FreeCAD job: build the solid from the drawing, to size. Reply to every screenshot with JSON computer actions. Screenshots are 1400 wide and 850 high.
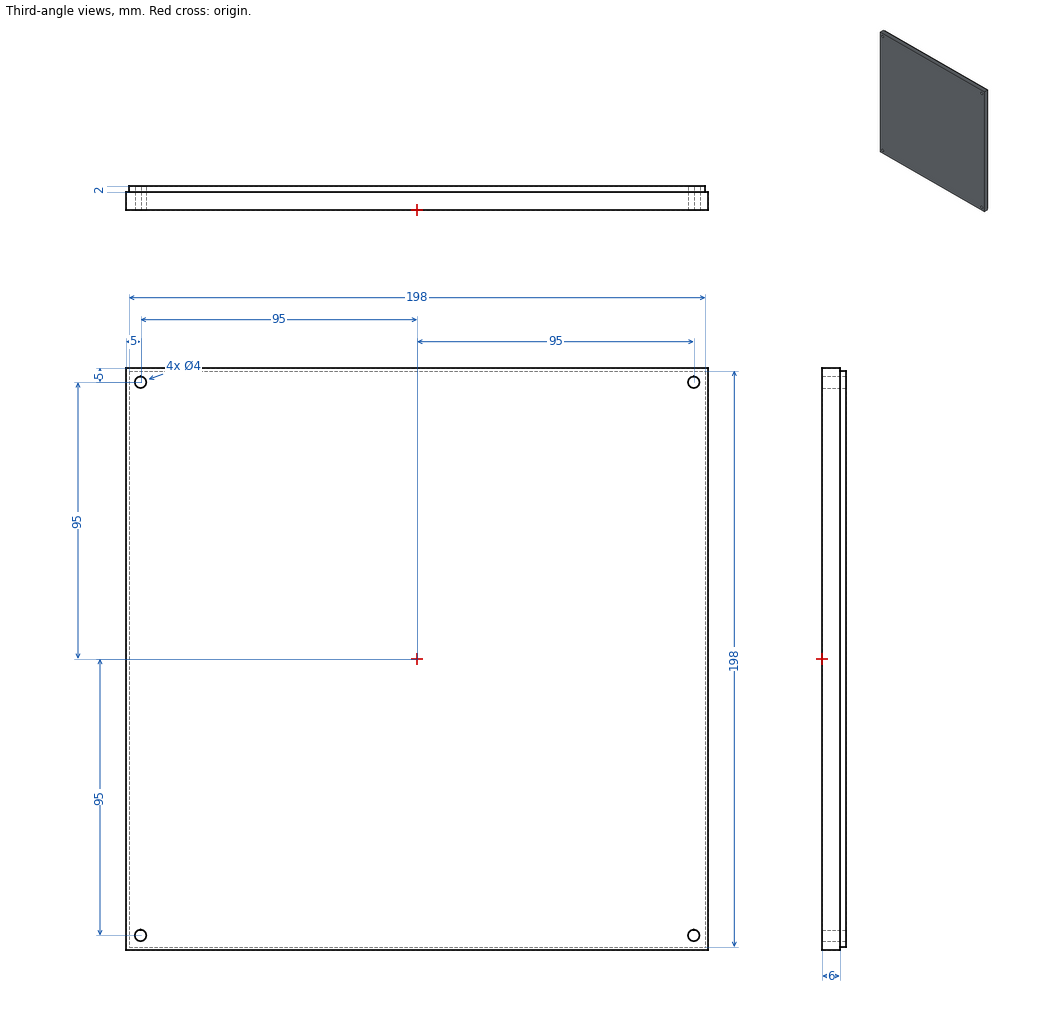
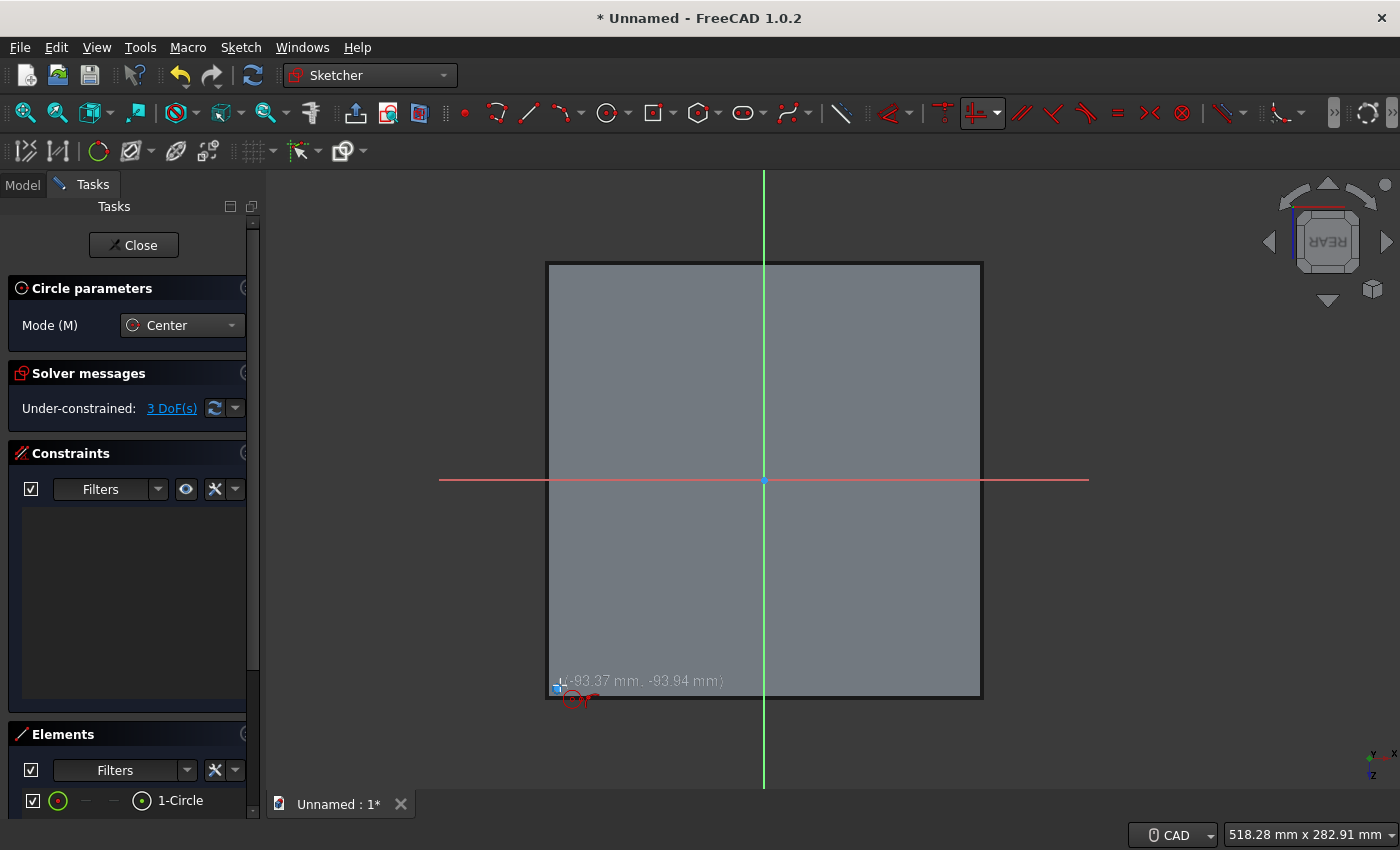
{"action": "scroll", "coordinate": [972, 688], "scroll_direction": "up", "scroll_amount": 9}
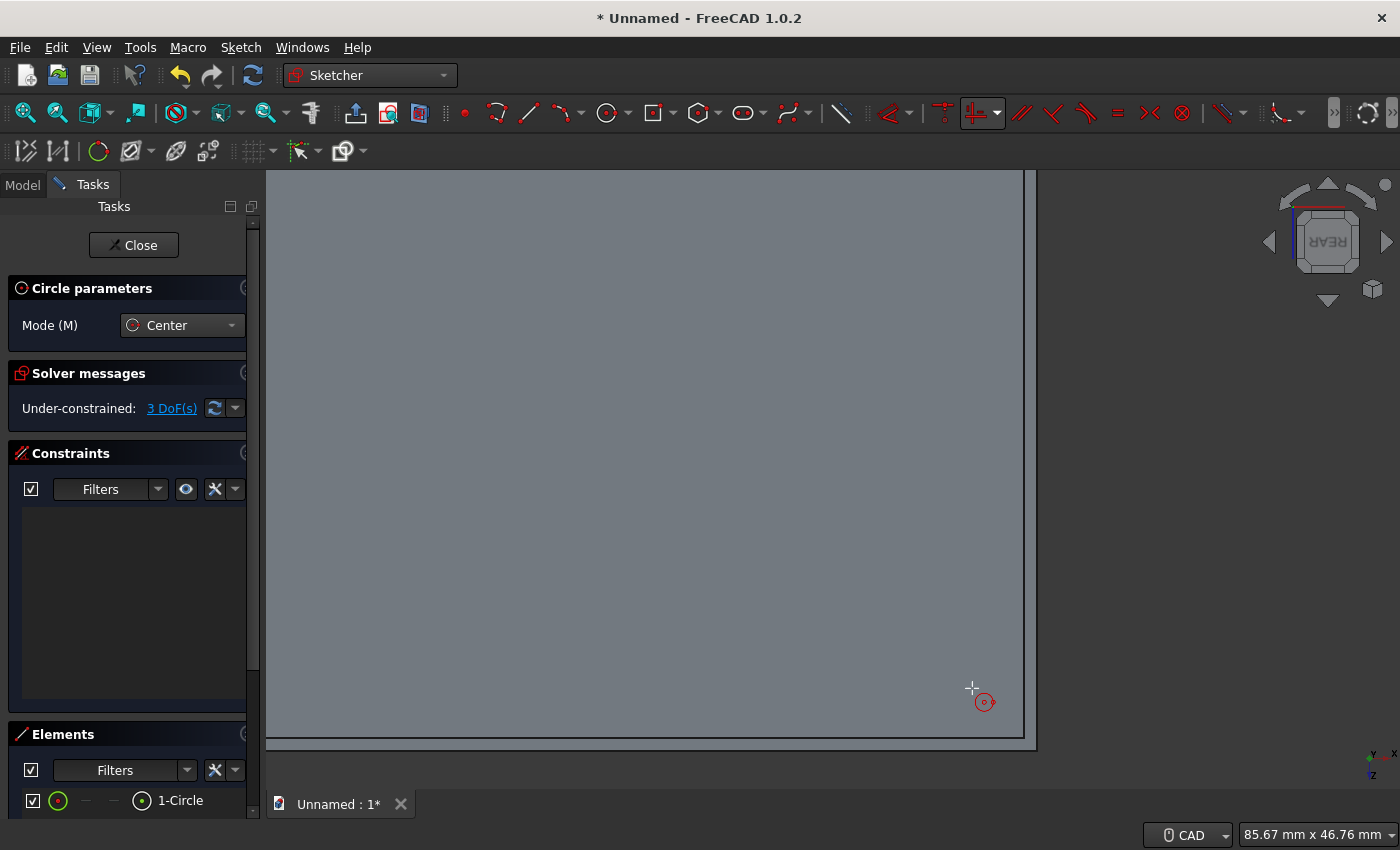
{"action": "scroll", "coordinate": [973, 688], "scroll_direction": "down", "scroll_amount": 9}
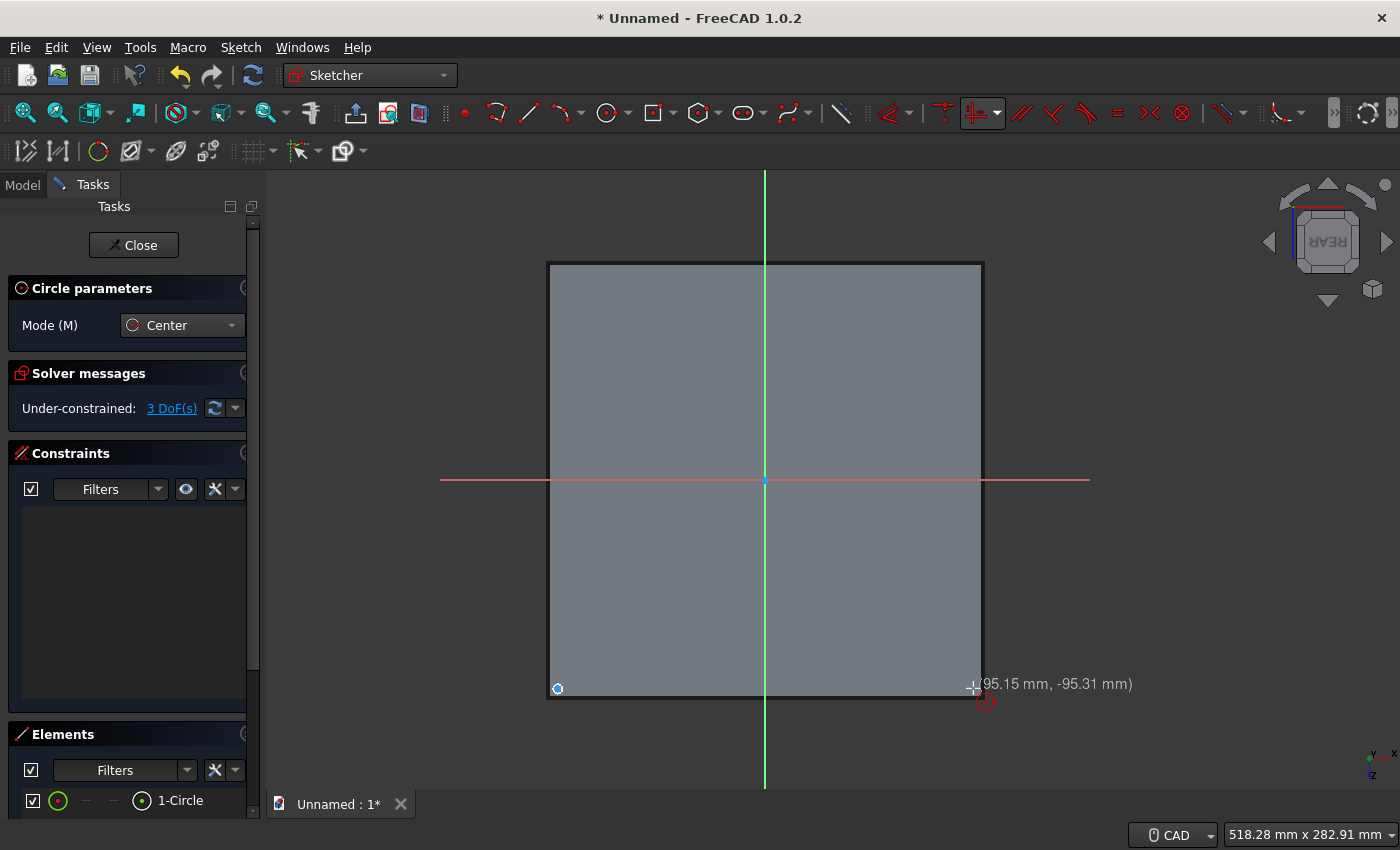
{"action": "left_click", "coordinate": [973, 688]}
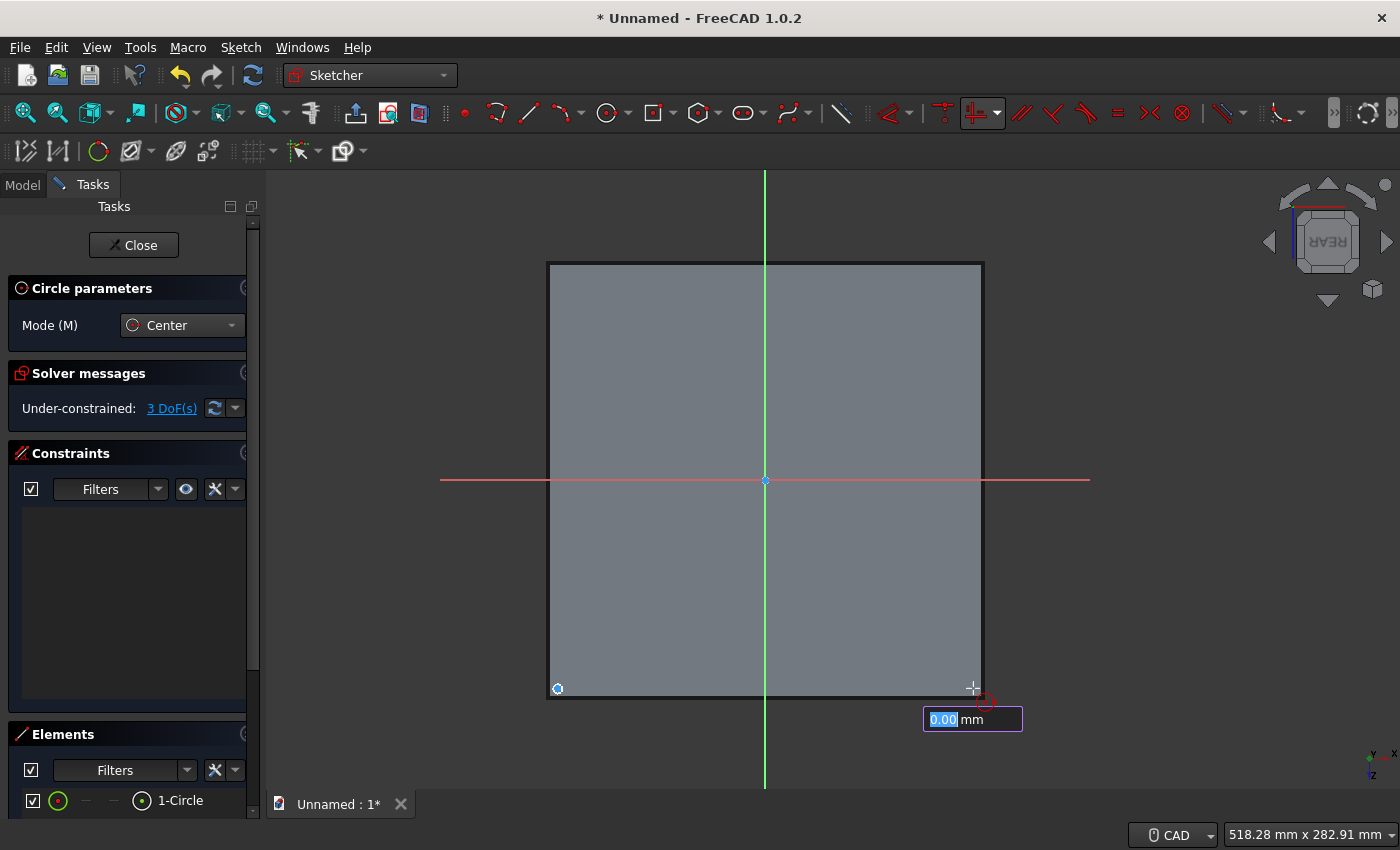
{"action": "scroll", "coordinate": [976, 685], "scroll_direction": "up", "scroll_amount": 7}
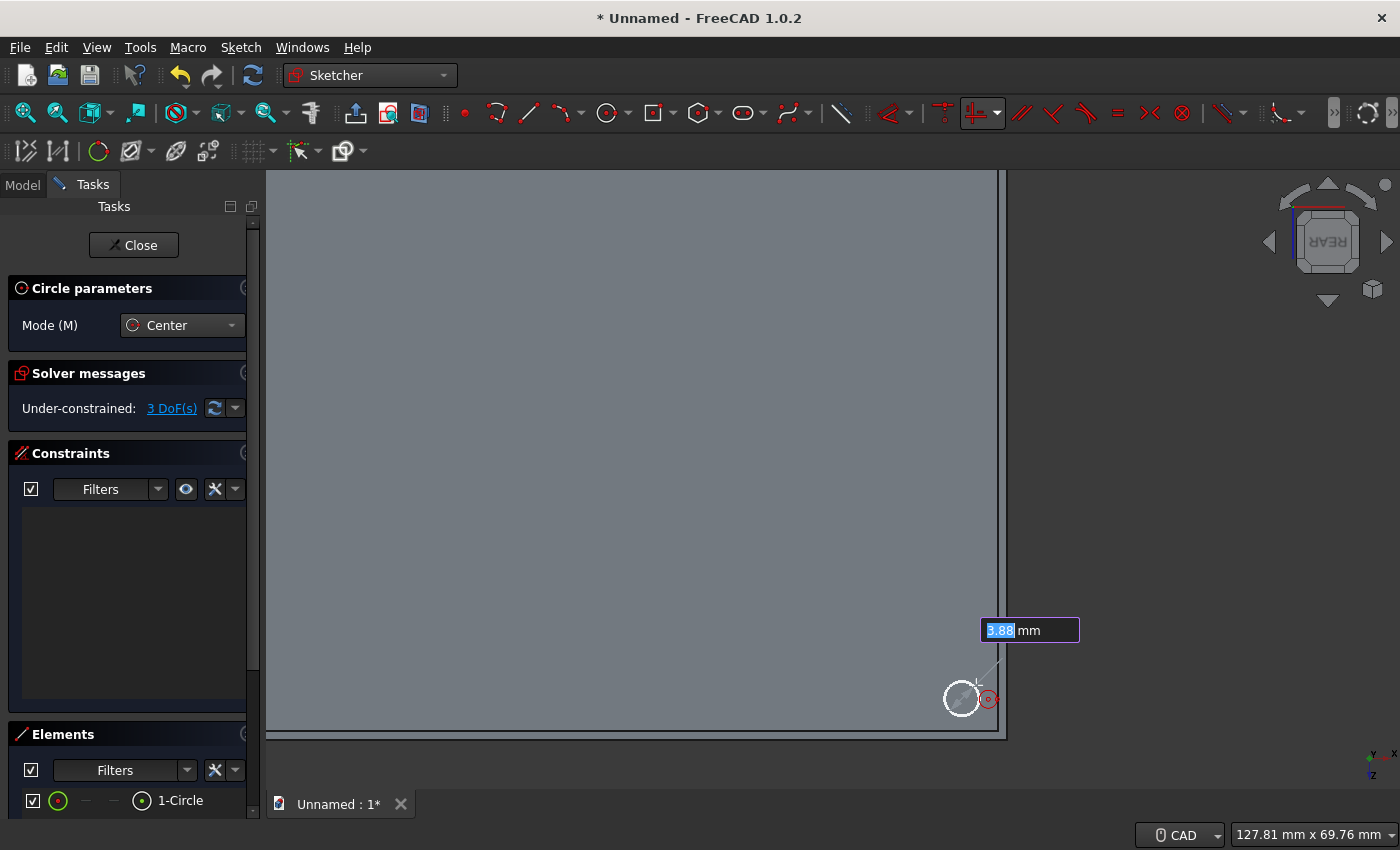
{"action": "left_click", "coordinate": [975, 683]}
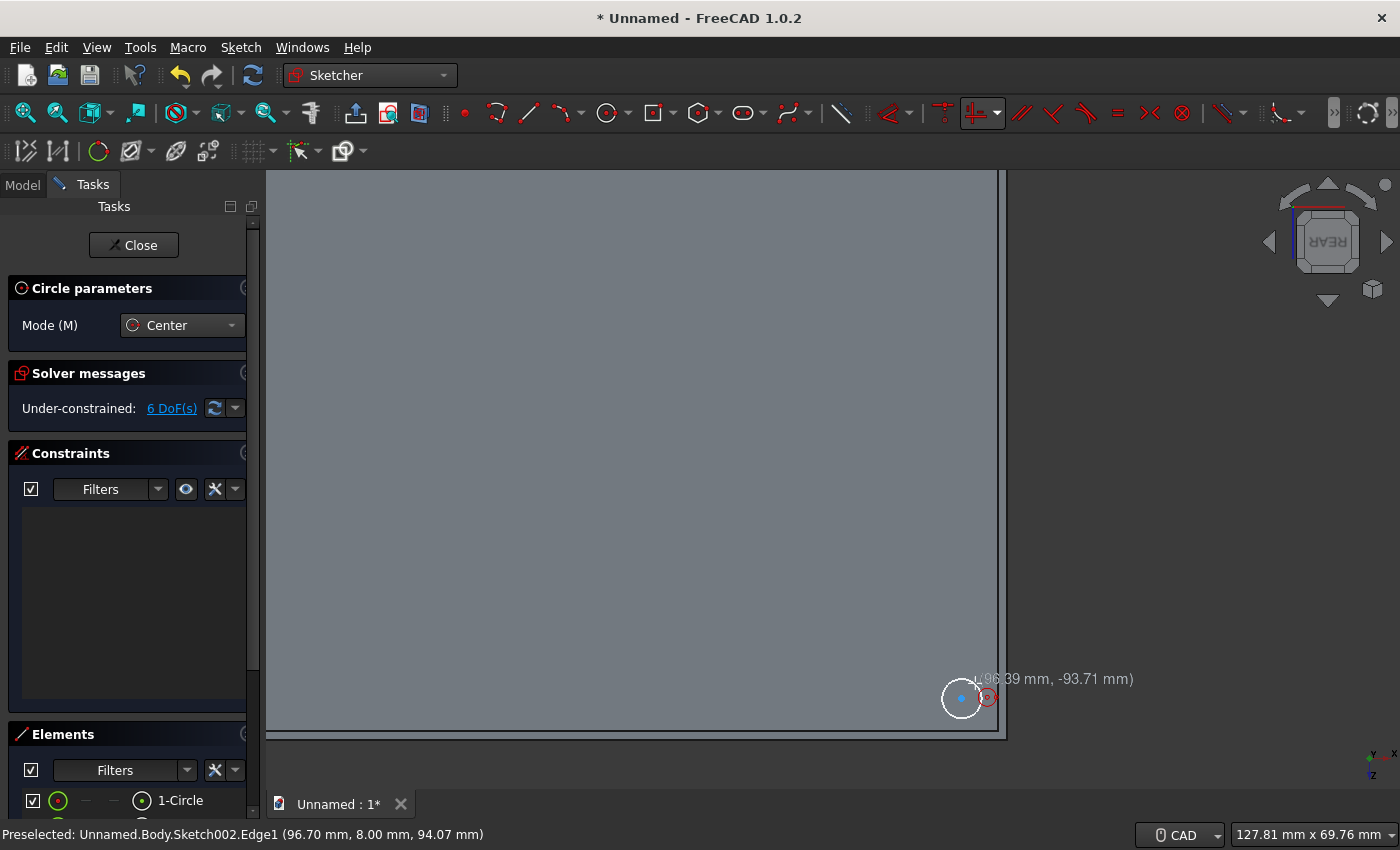
{"action": "scroll", "coordinate": [976, 685], "scroll_direction": "down", "scroll_amount": 7}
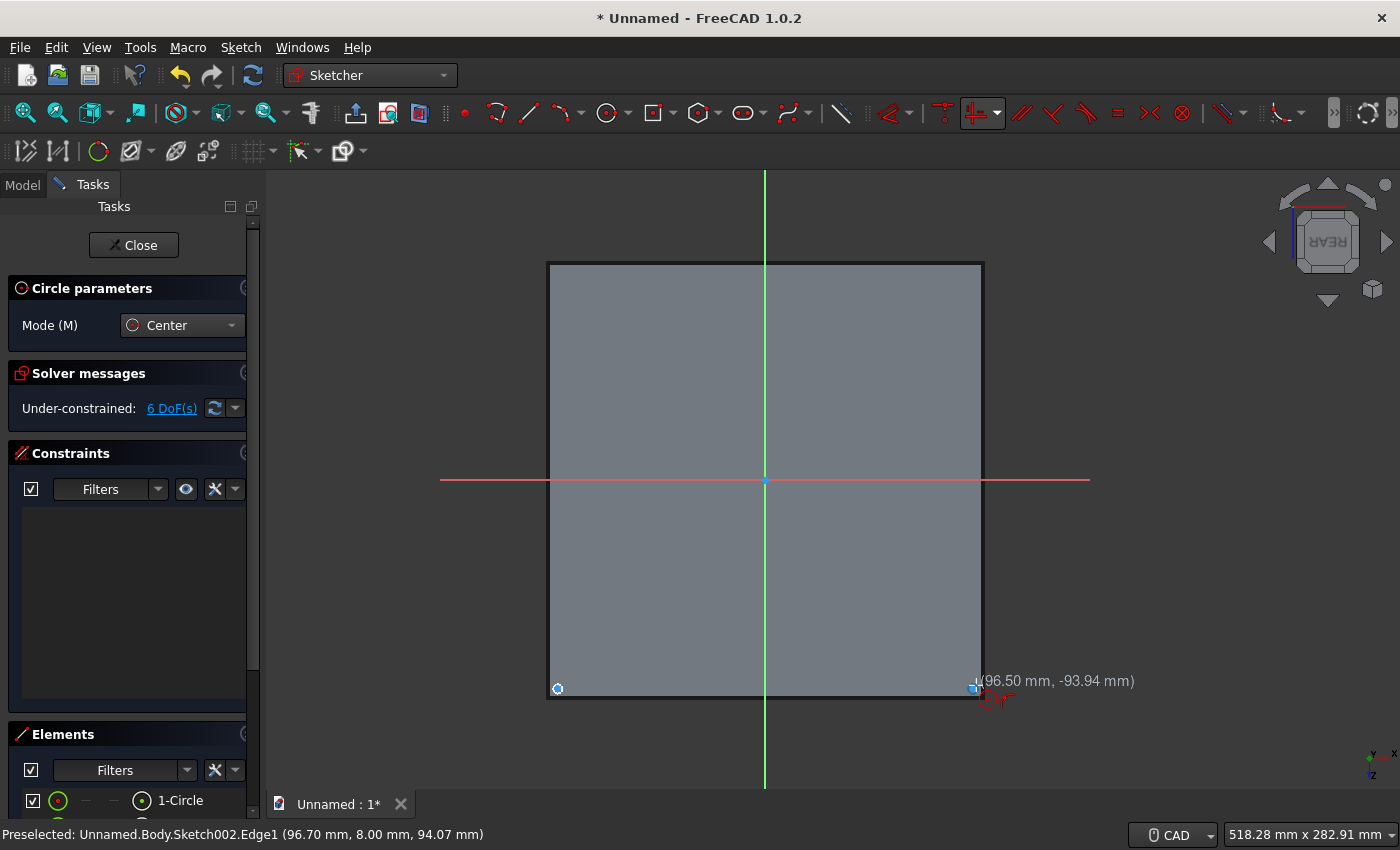
{"action": "scroll", "coordinate": [973, 272], "scroll_direction": "up", "scroll_amount": 9}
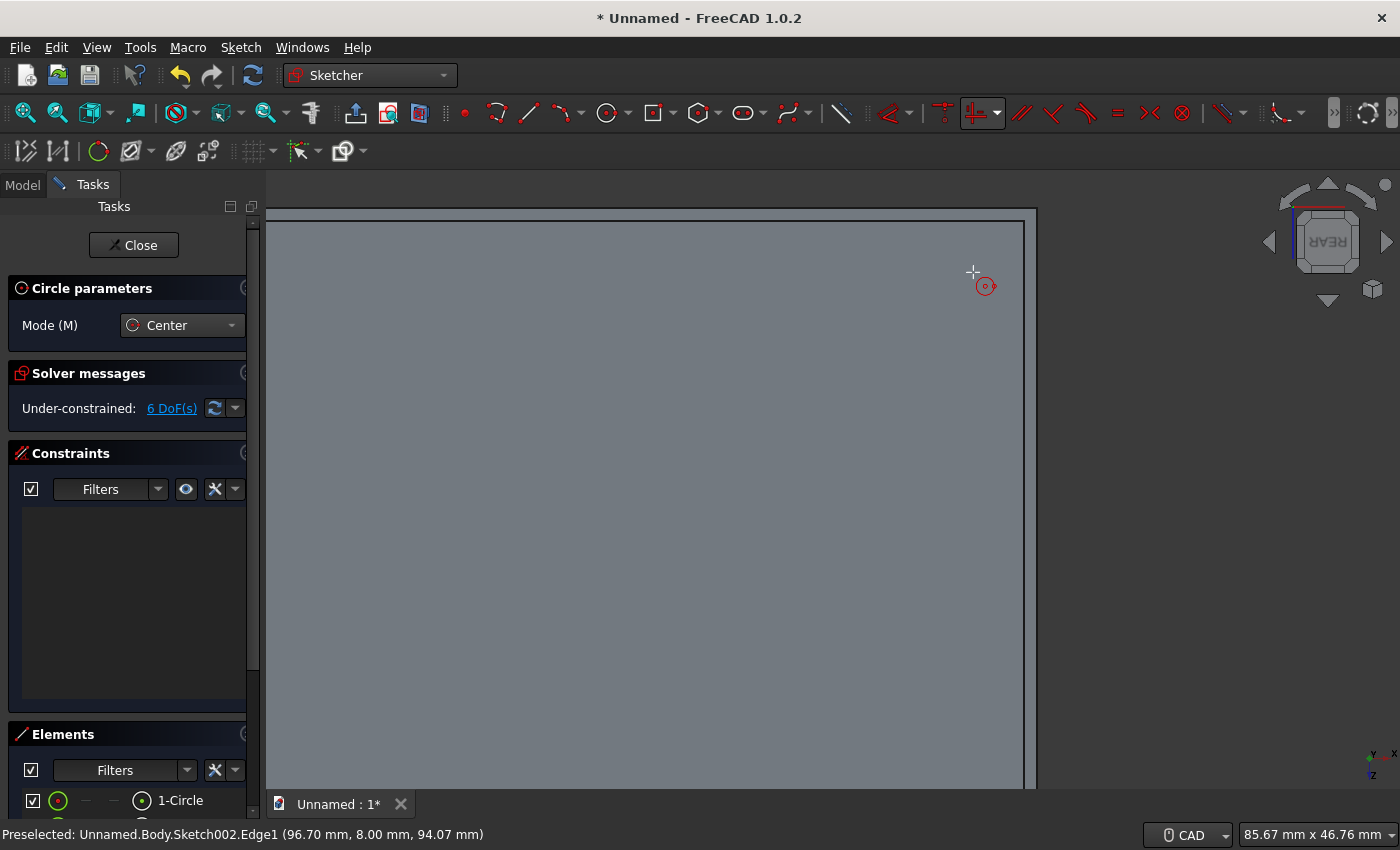
{"action": "scroll", "coordinate": [973, 271], "scroll_direction": "down", "scroll_amount": 9}